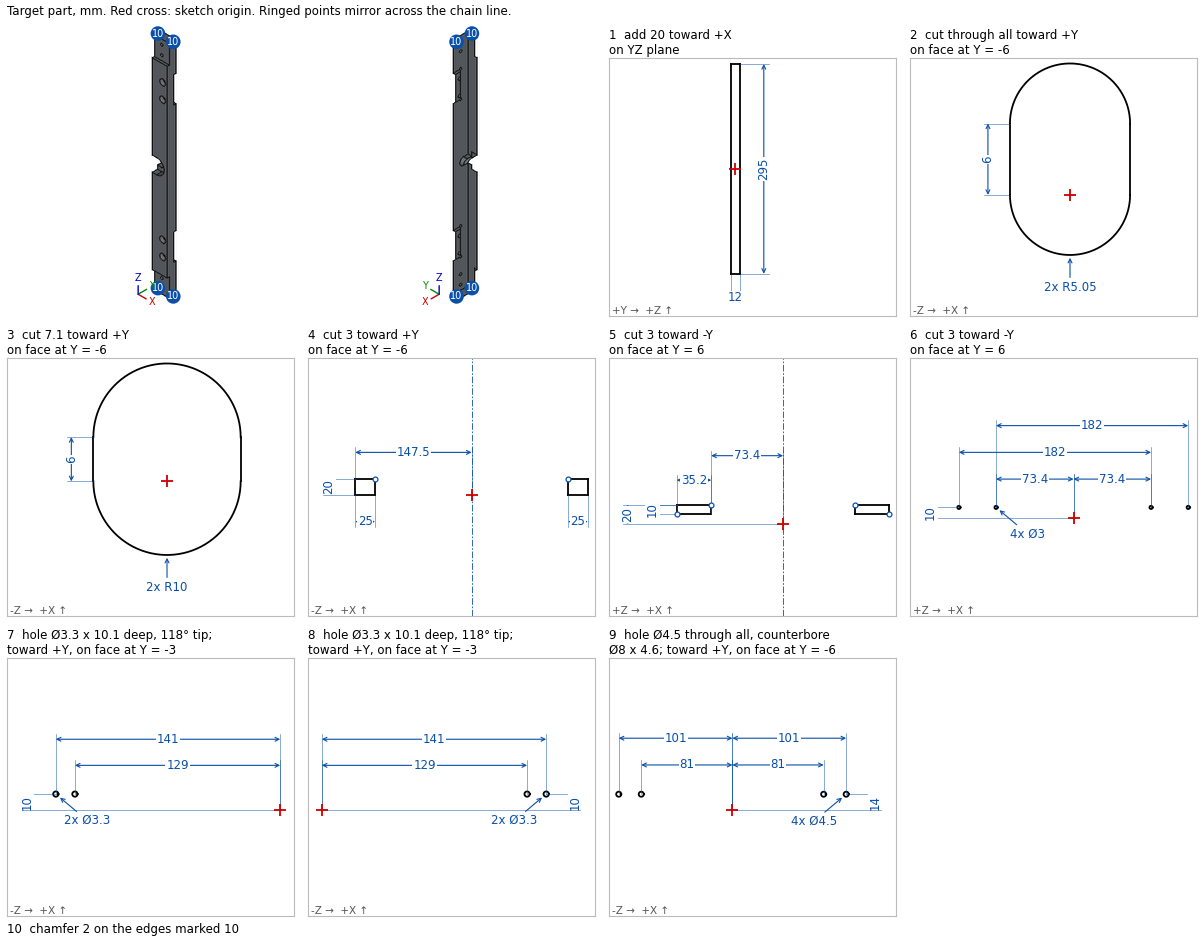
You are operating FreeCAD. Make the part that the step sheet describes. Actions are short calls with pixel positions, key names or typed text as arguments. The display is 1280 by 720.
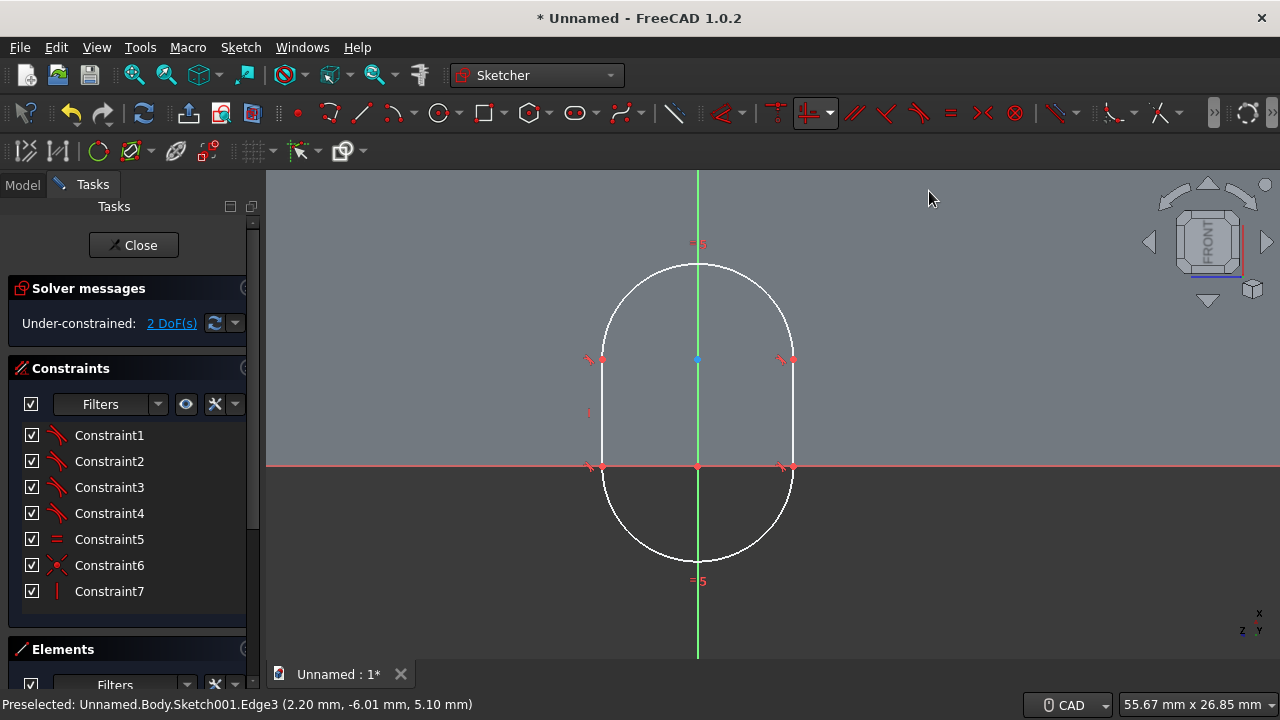
click(722, 114)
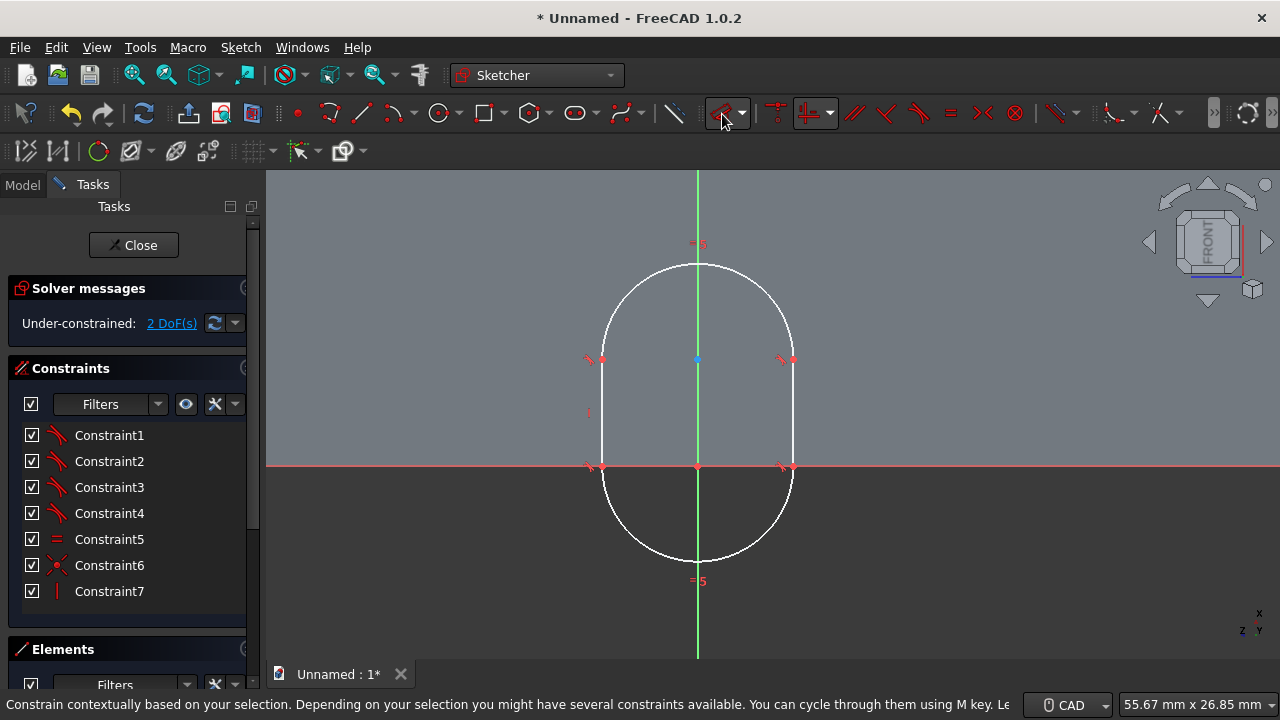
click(642, 543)
click(623, 569)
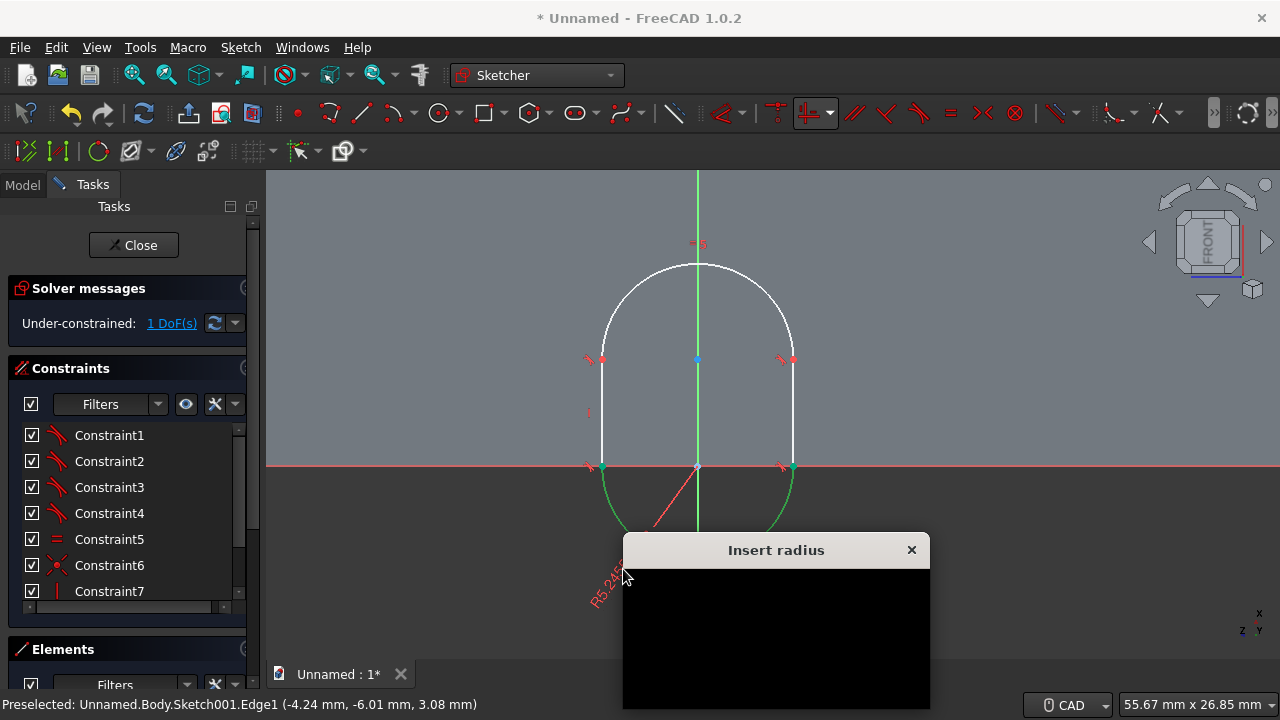
text(5.05)
key(Return)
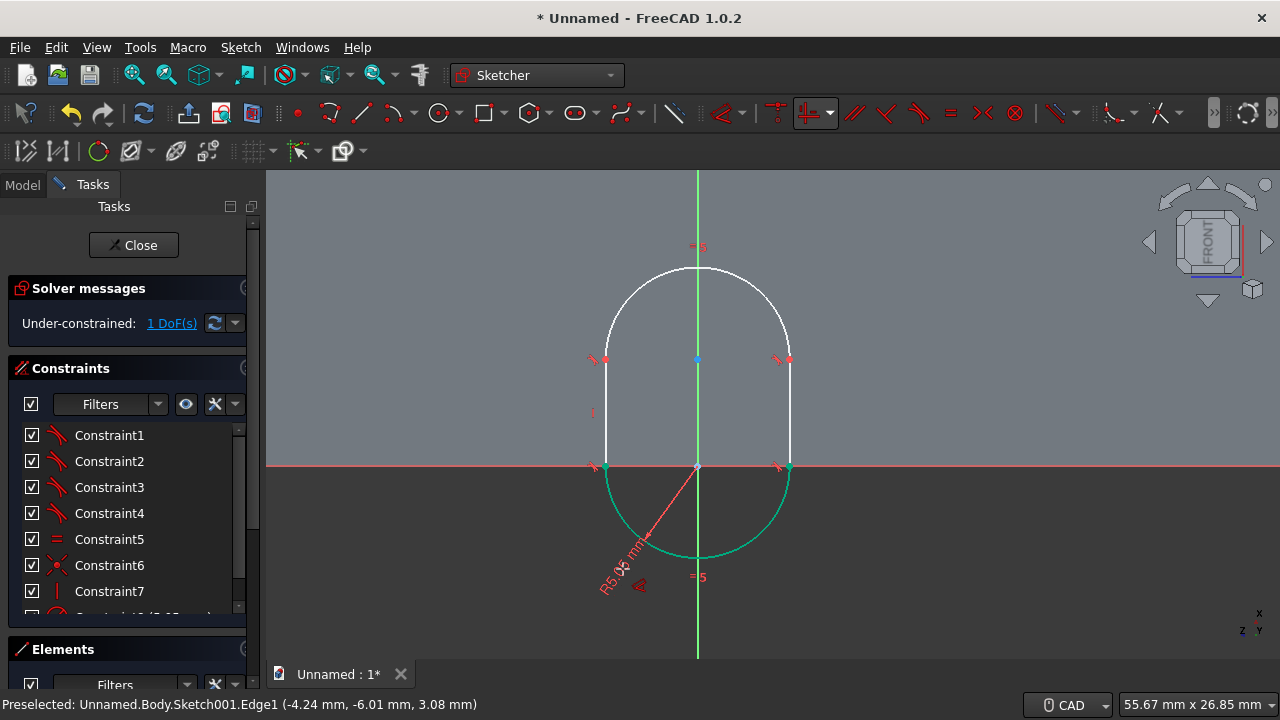
click(606, 434)
click(572, 413)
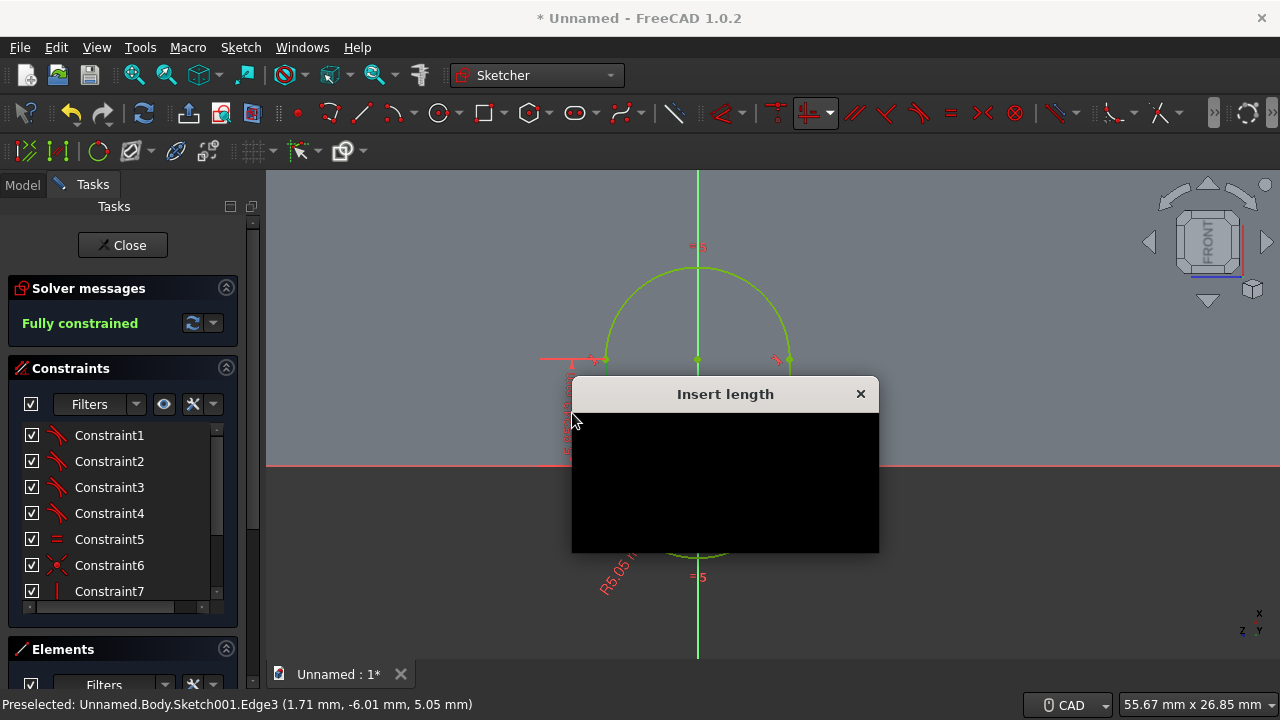
text(6)
key(Return)
key(Escape)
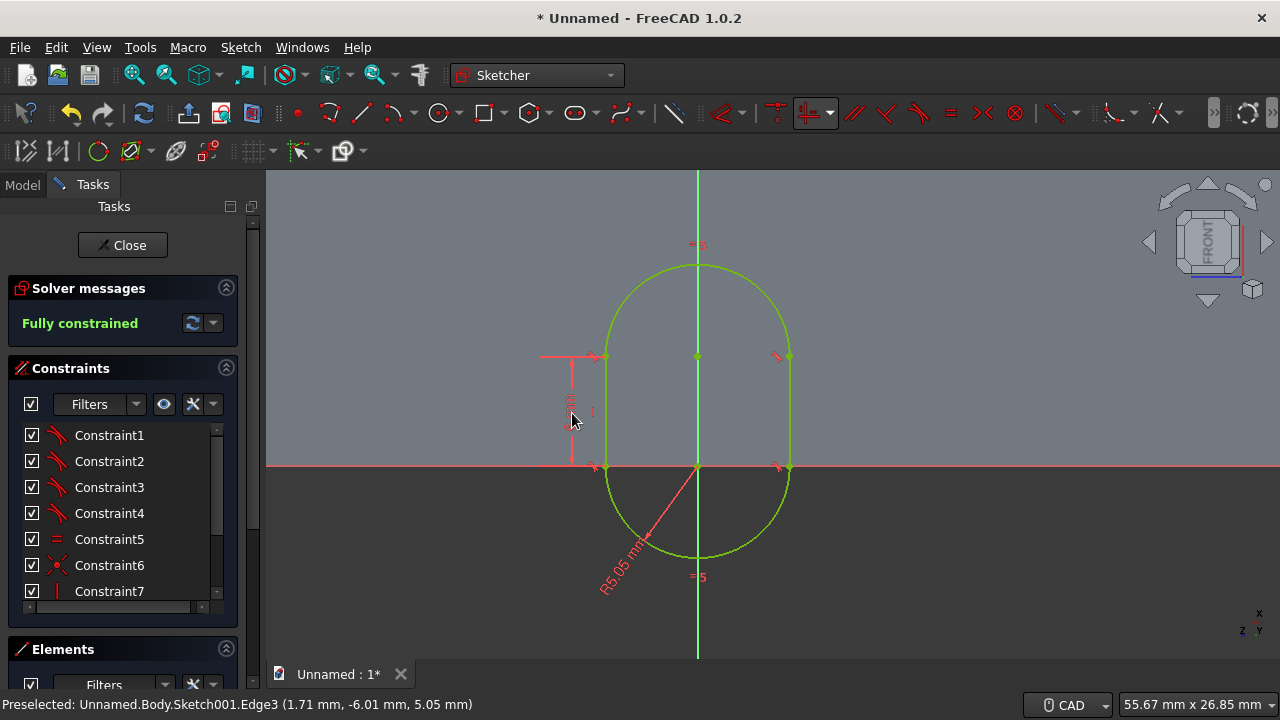
click(123, 245)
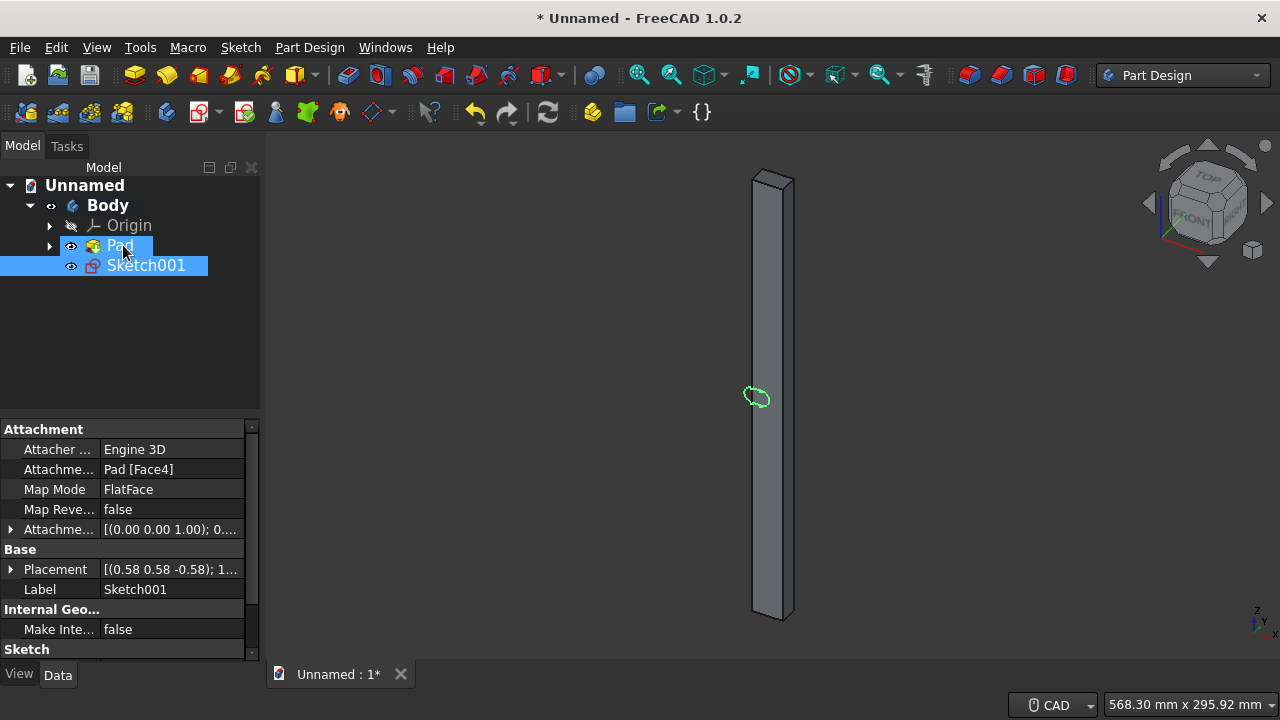
click(350, 76)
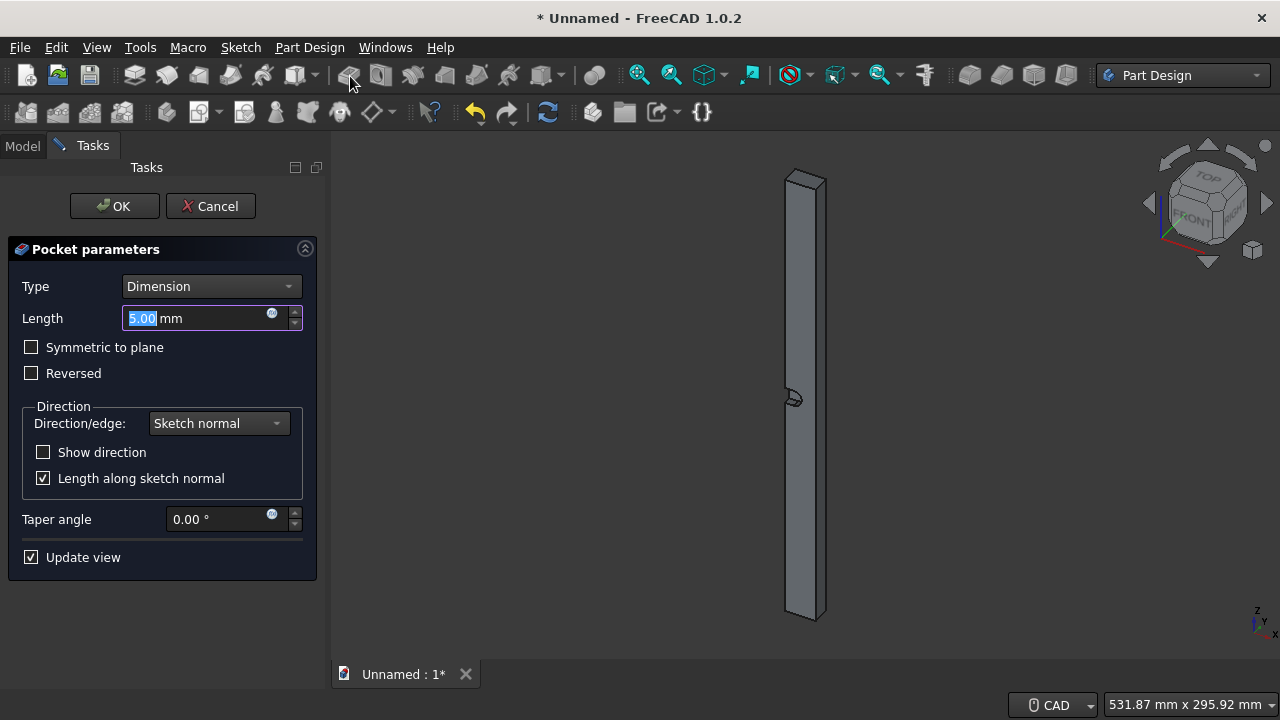
click(212, 286)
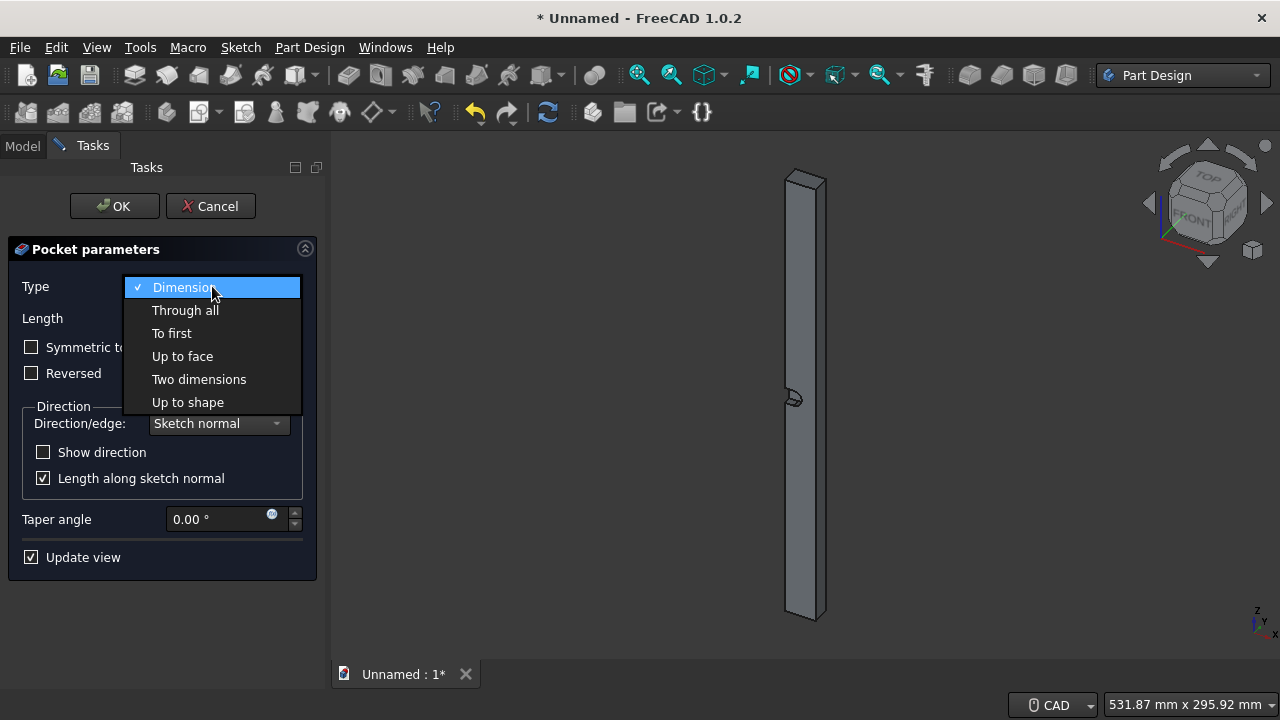
click(212, 310)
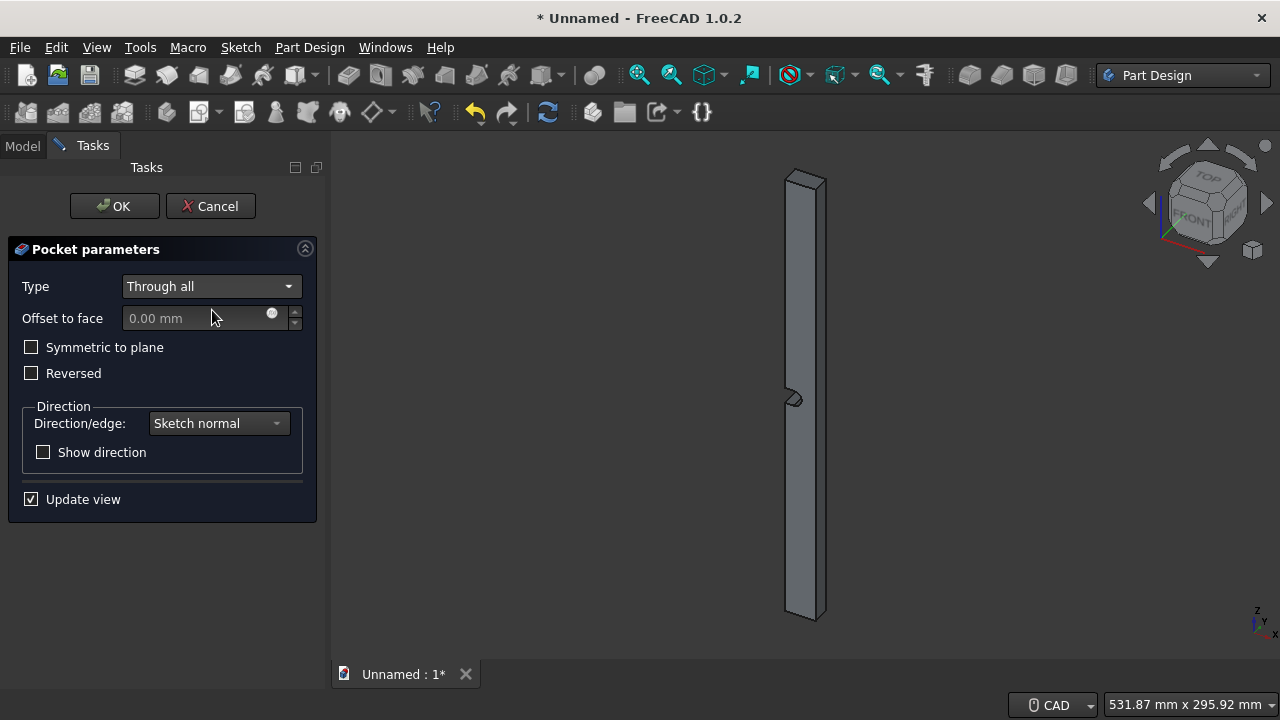
click(115, 206)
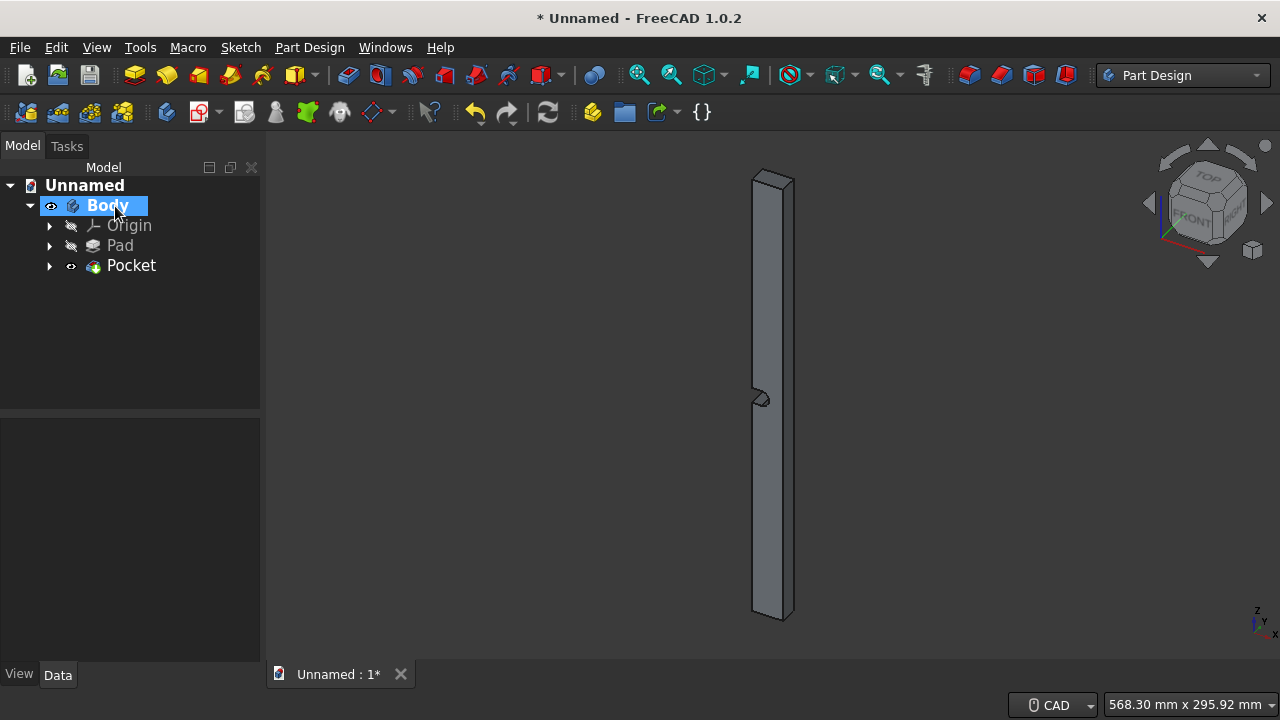
click(768, 461)